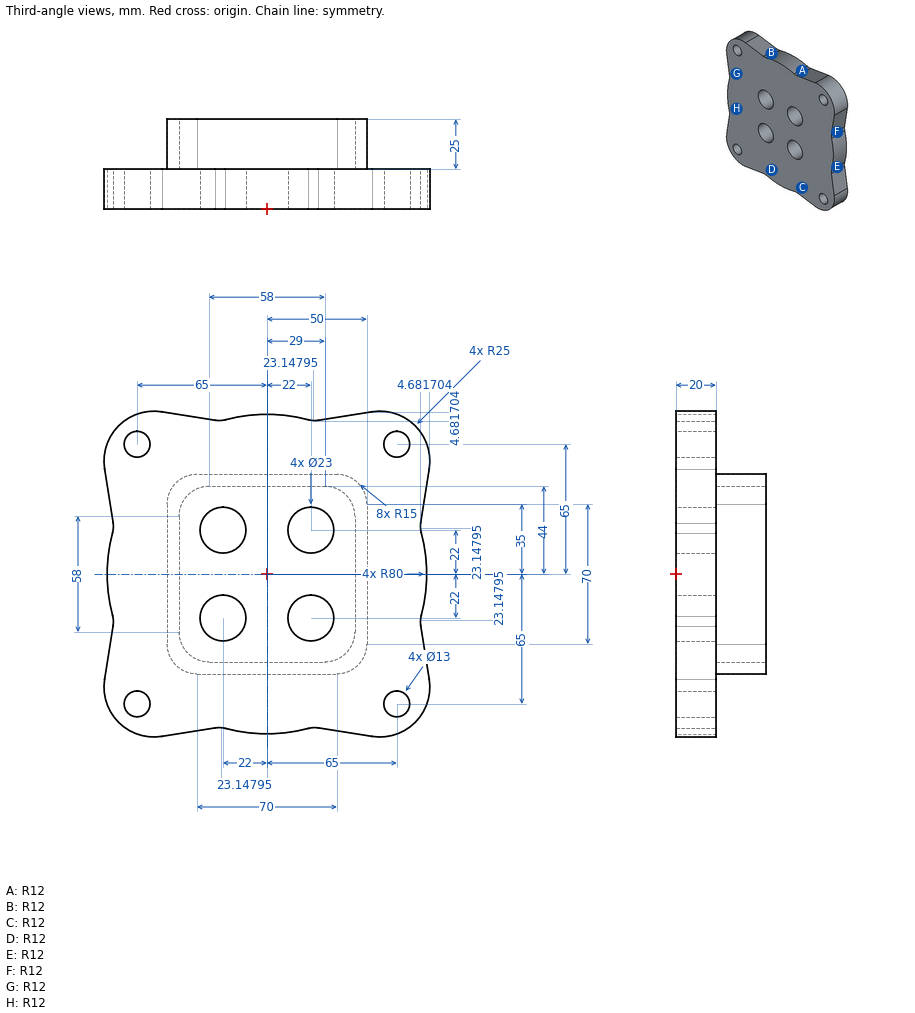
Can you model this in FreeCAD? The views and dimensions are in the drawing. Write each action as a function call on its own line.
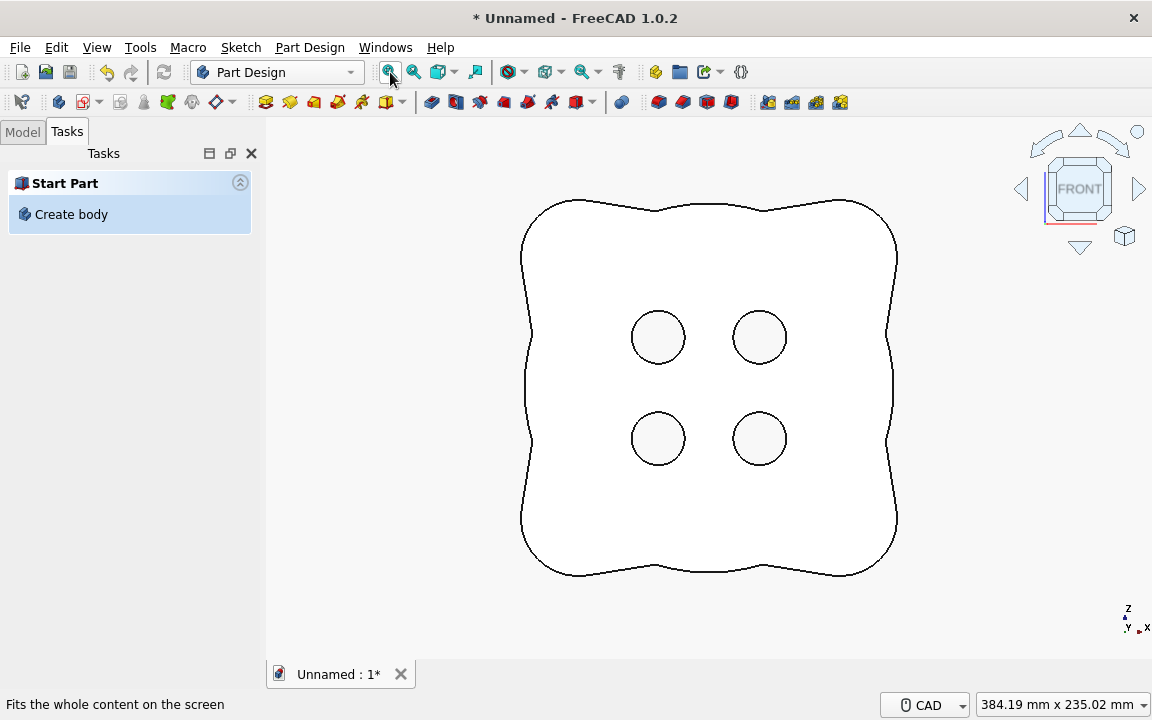
key(3)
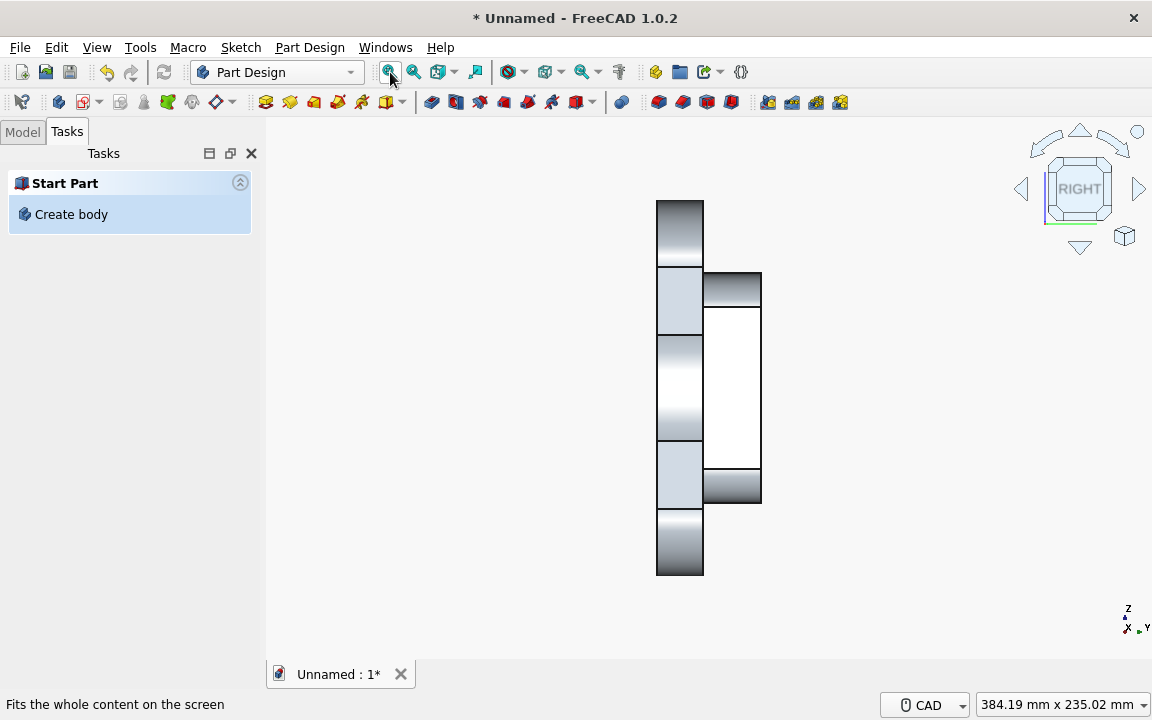
key(5)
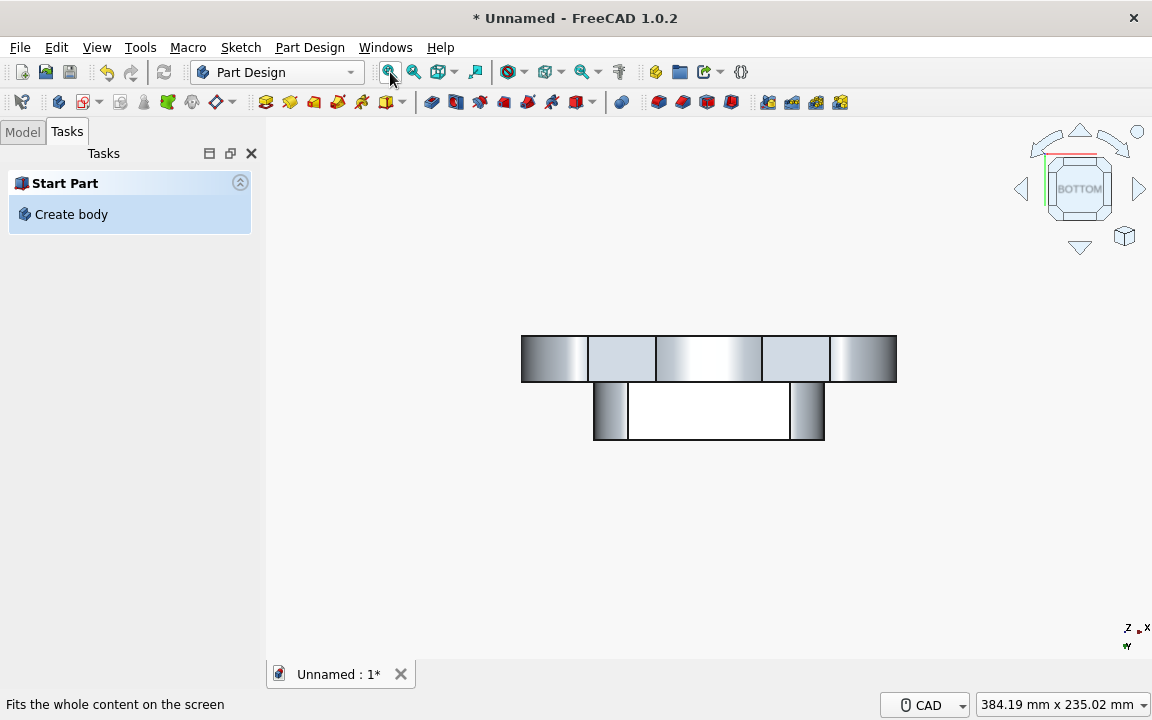
click(390, 72)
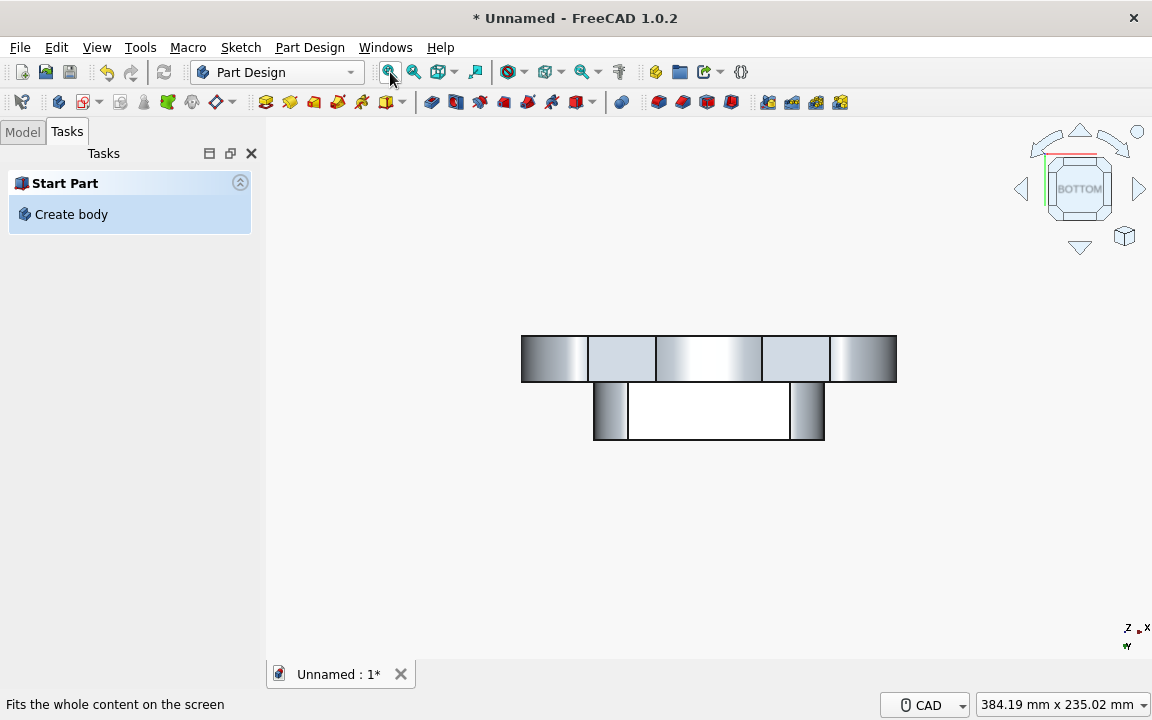
key(4)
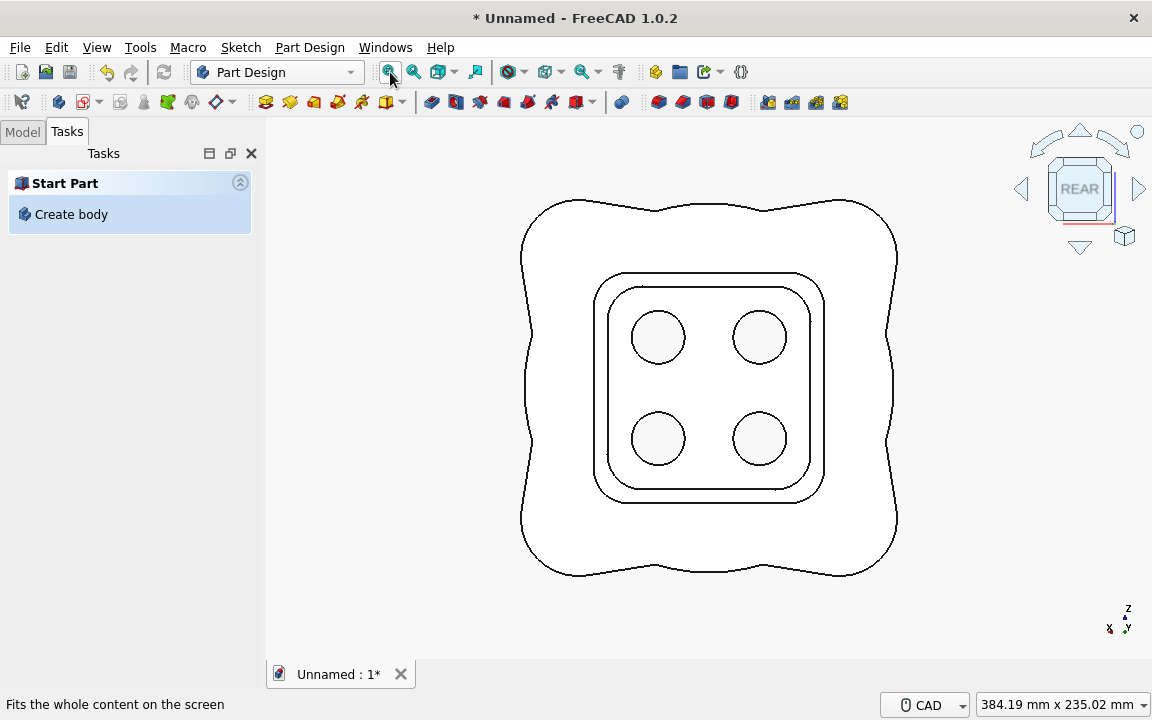
key(6)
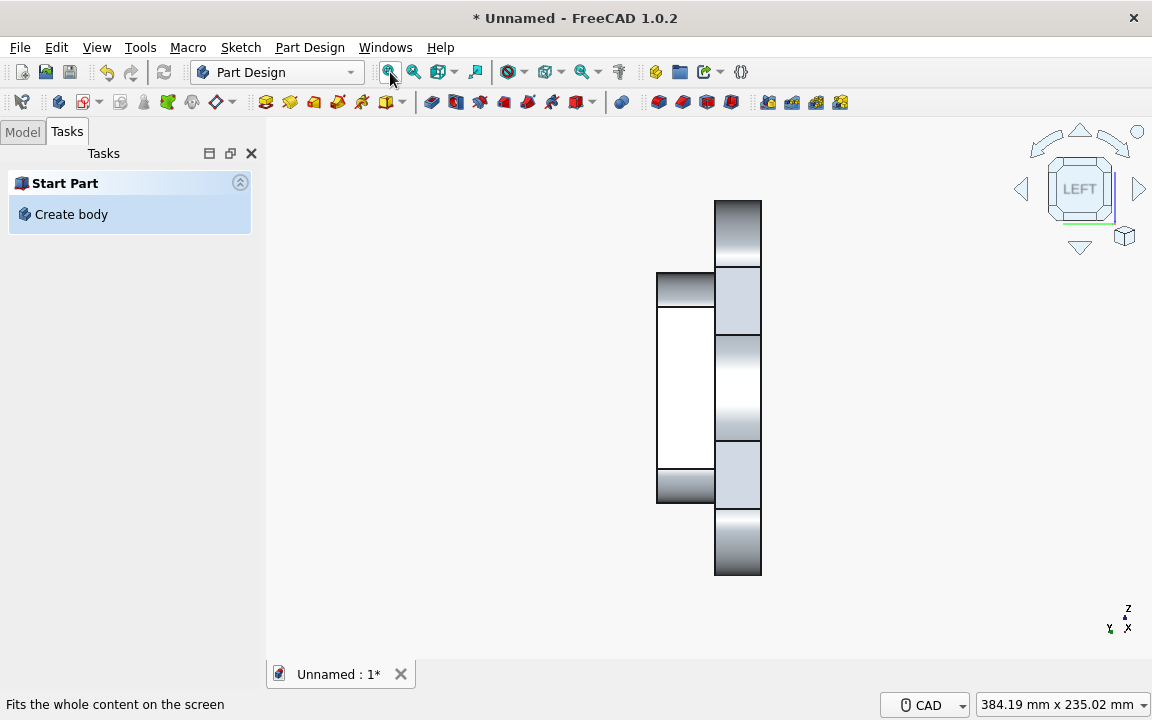
key(v)
key(3)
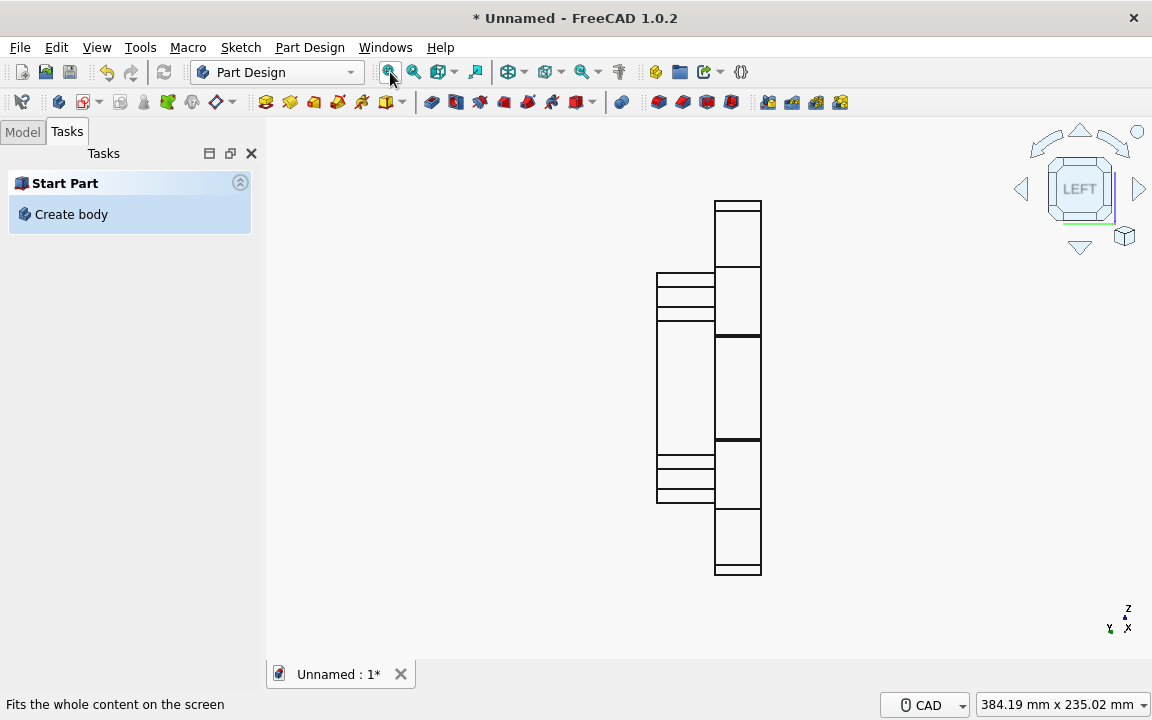
key(0)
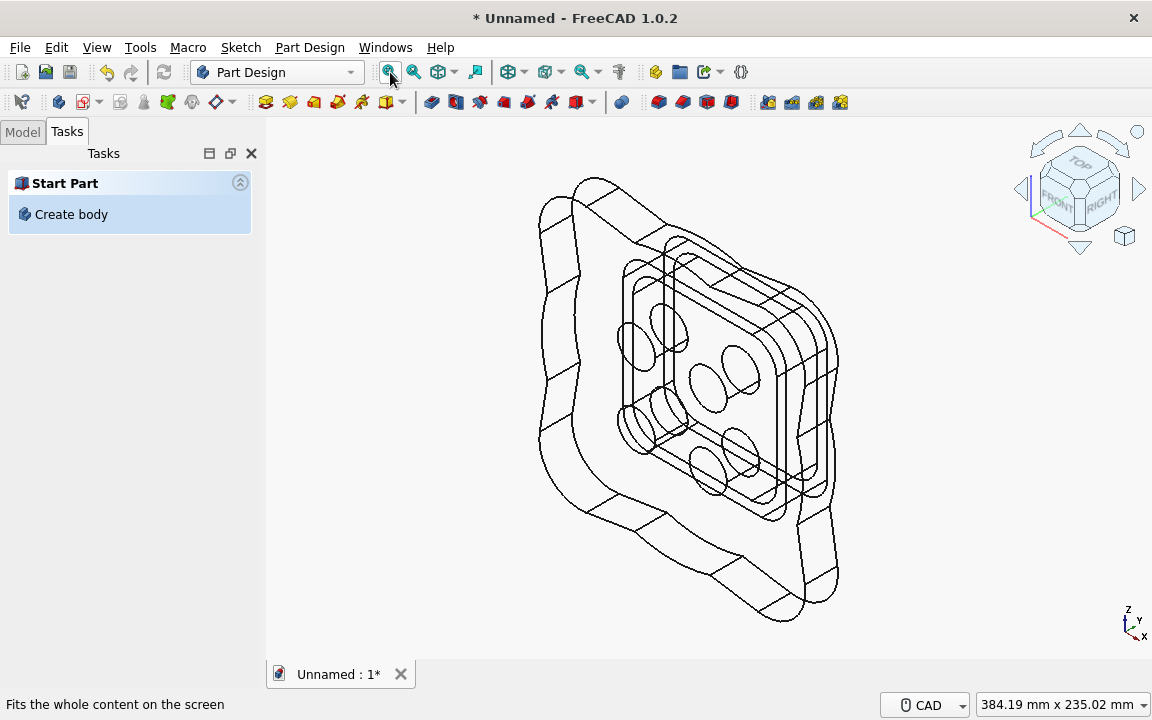
click(726, 276)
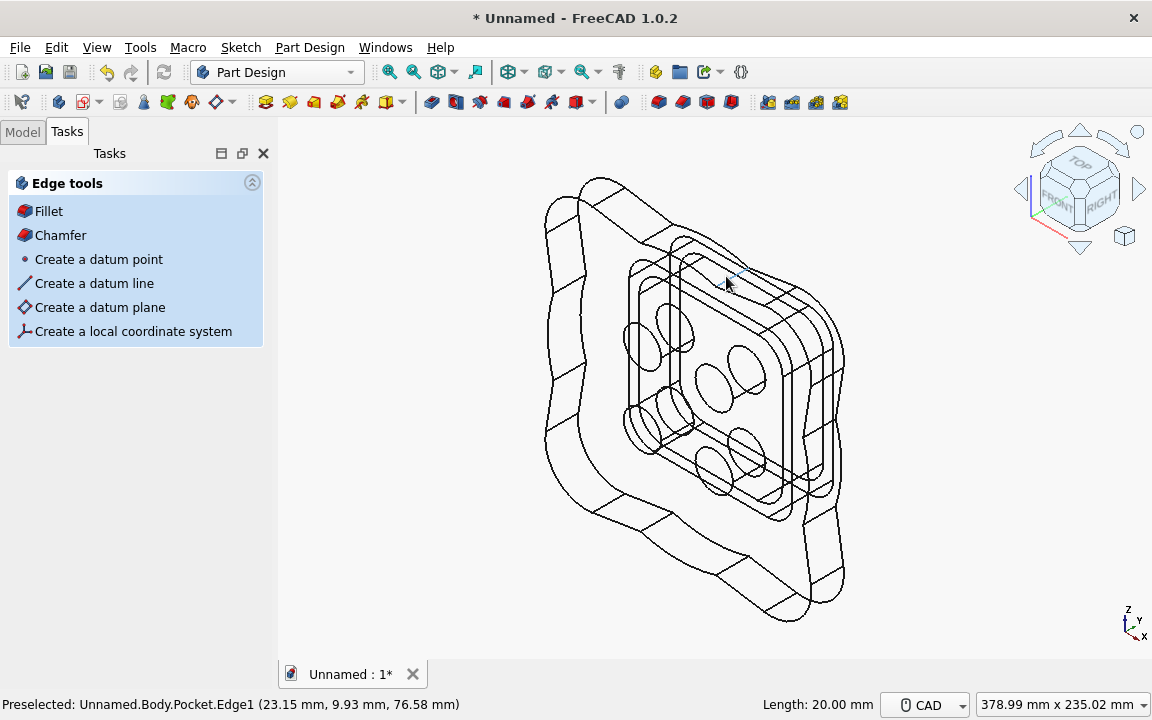
key(v)
key(1)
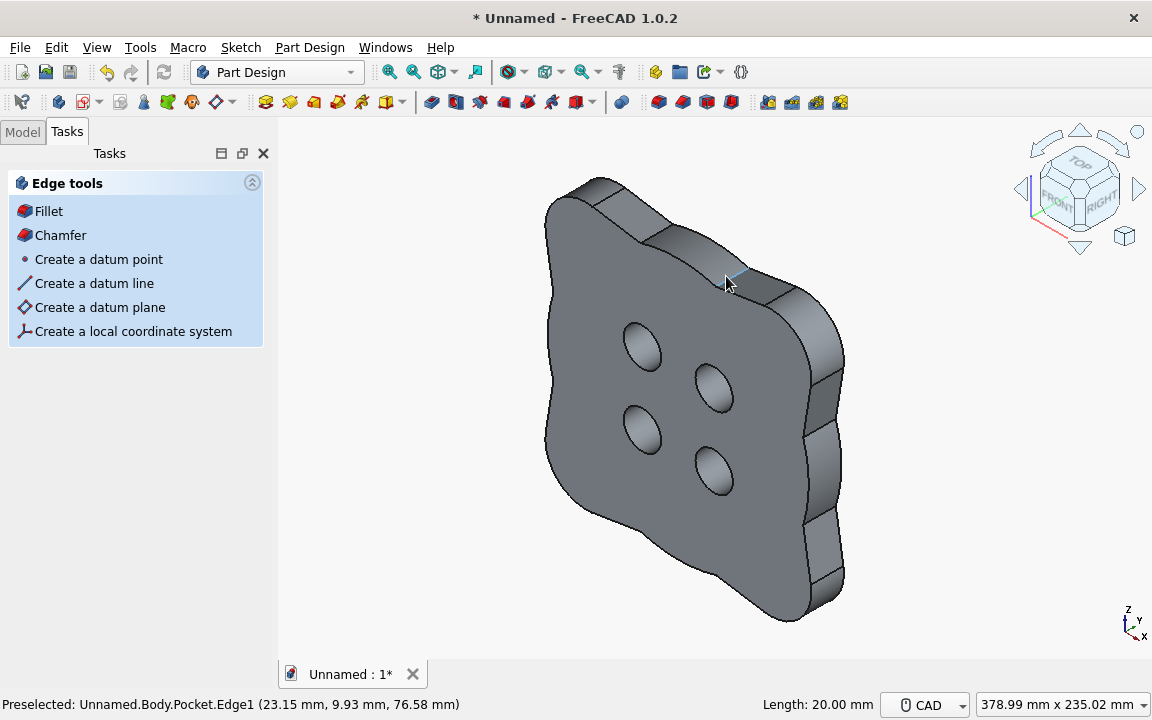
click(660, 102)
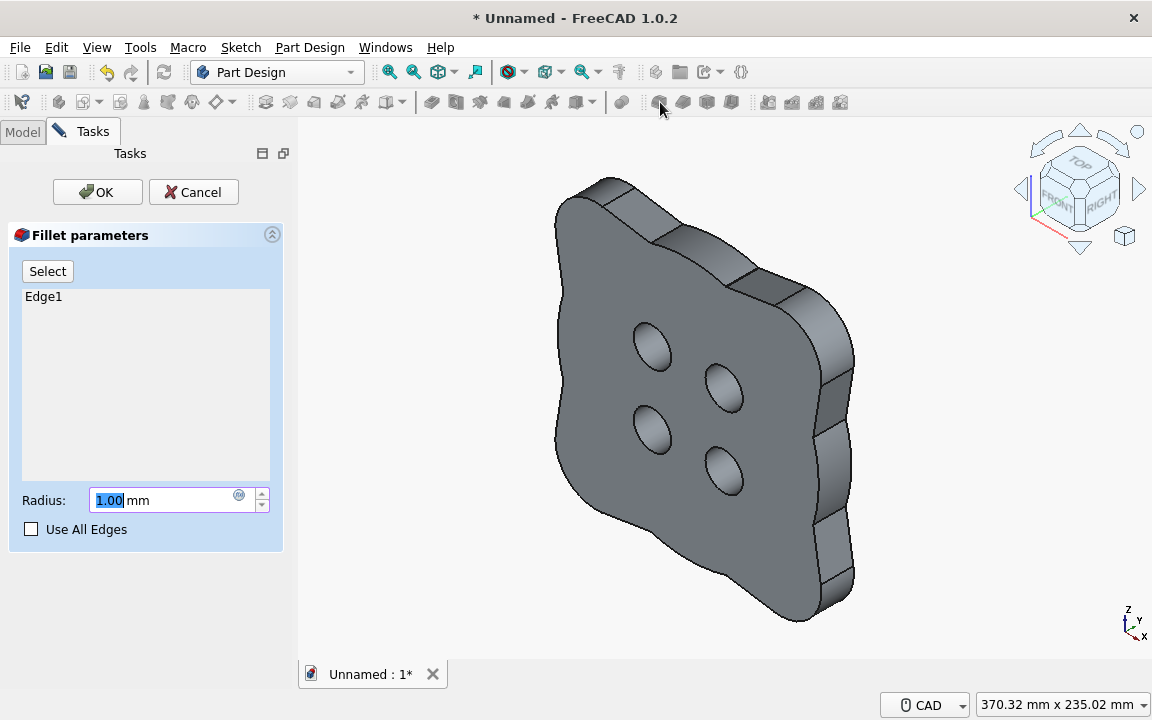
text(12)
key(Tab)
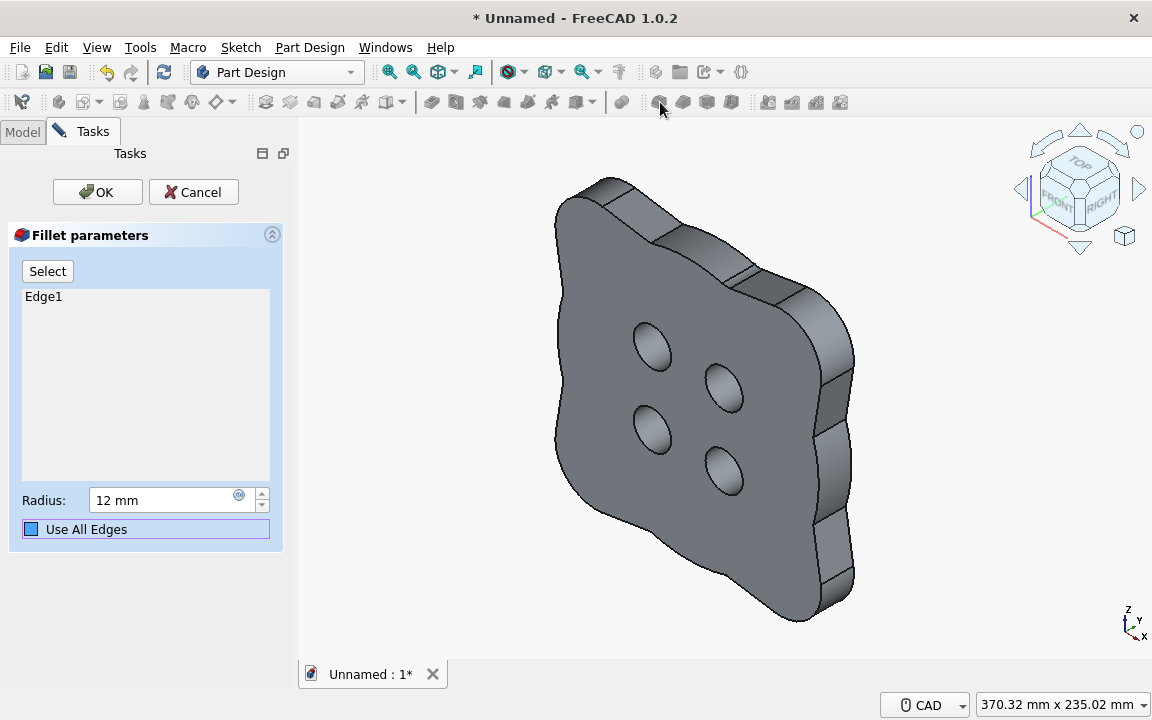
click(98, 192)